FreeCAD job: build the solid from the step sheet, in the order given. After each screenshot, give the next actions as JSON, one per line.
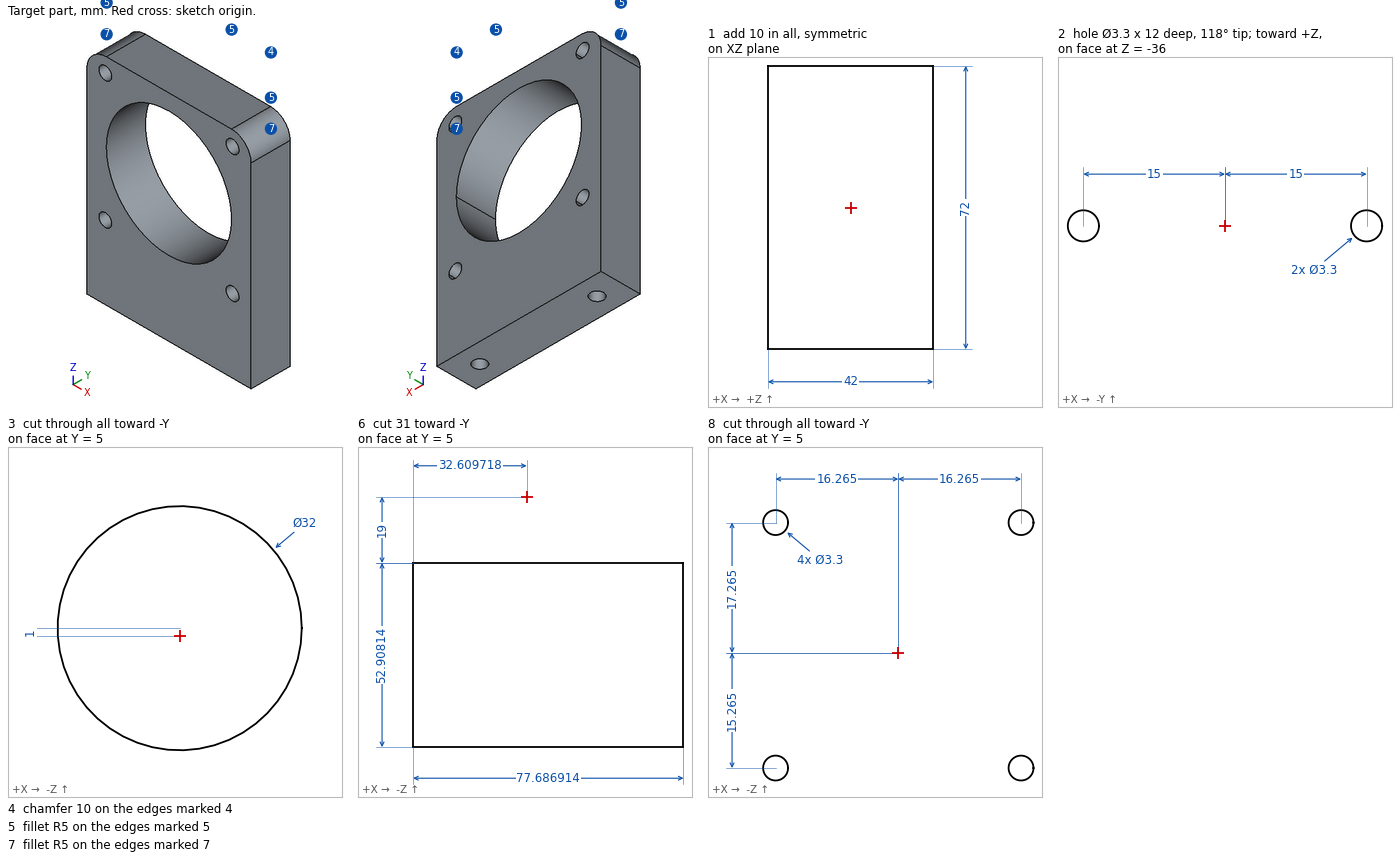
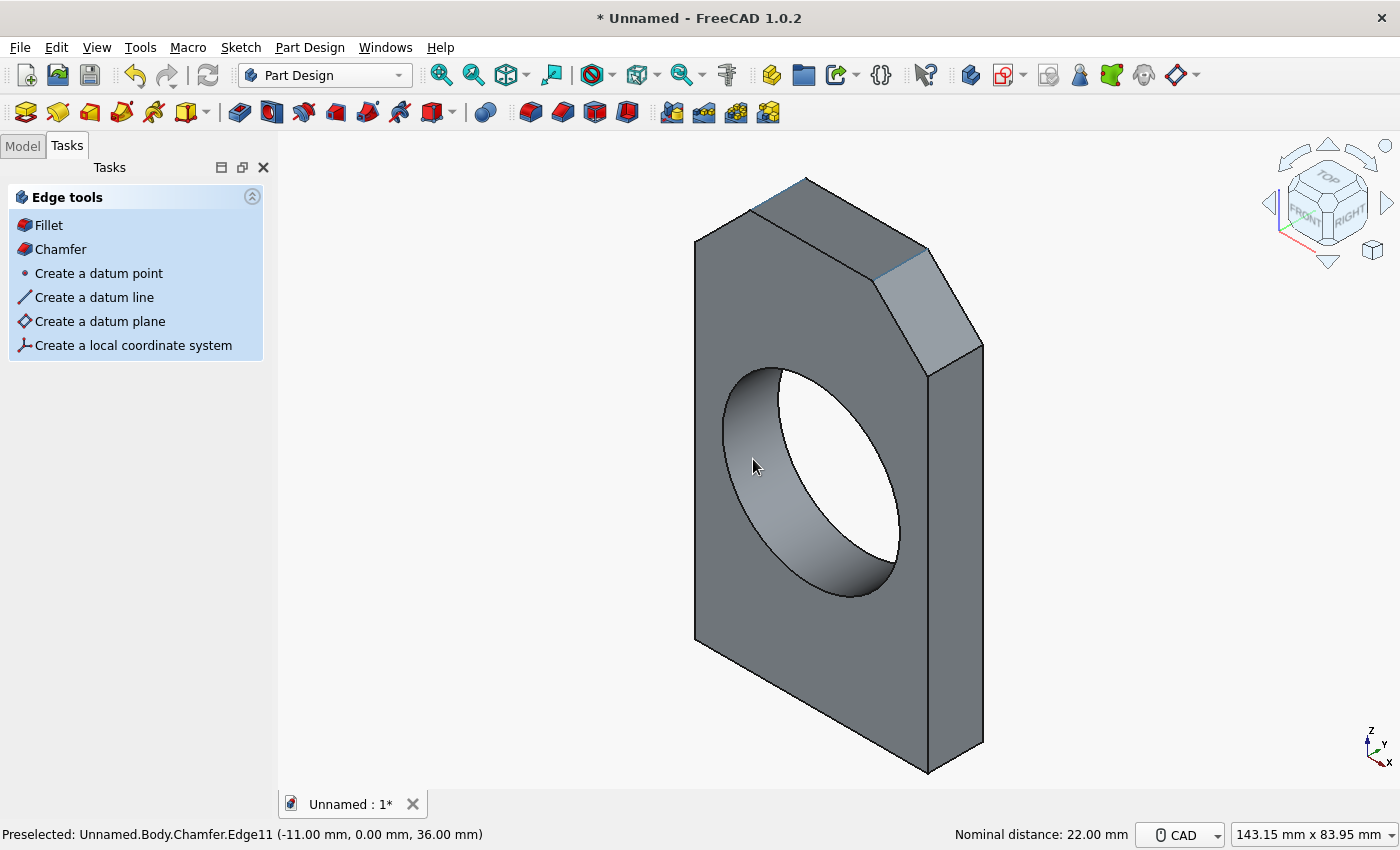
{"action": "left_click", "coordinate": [955, 360], "text": "ctrl"}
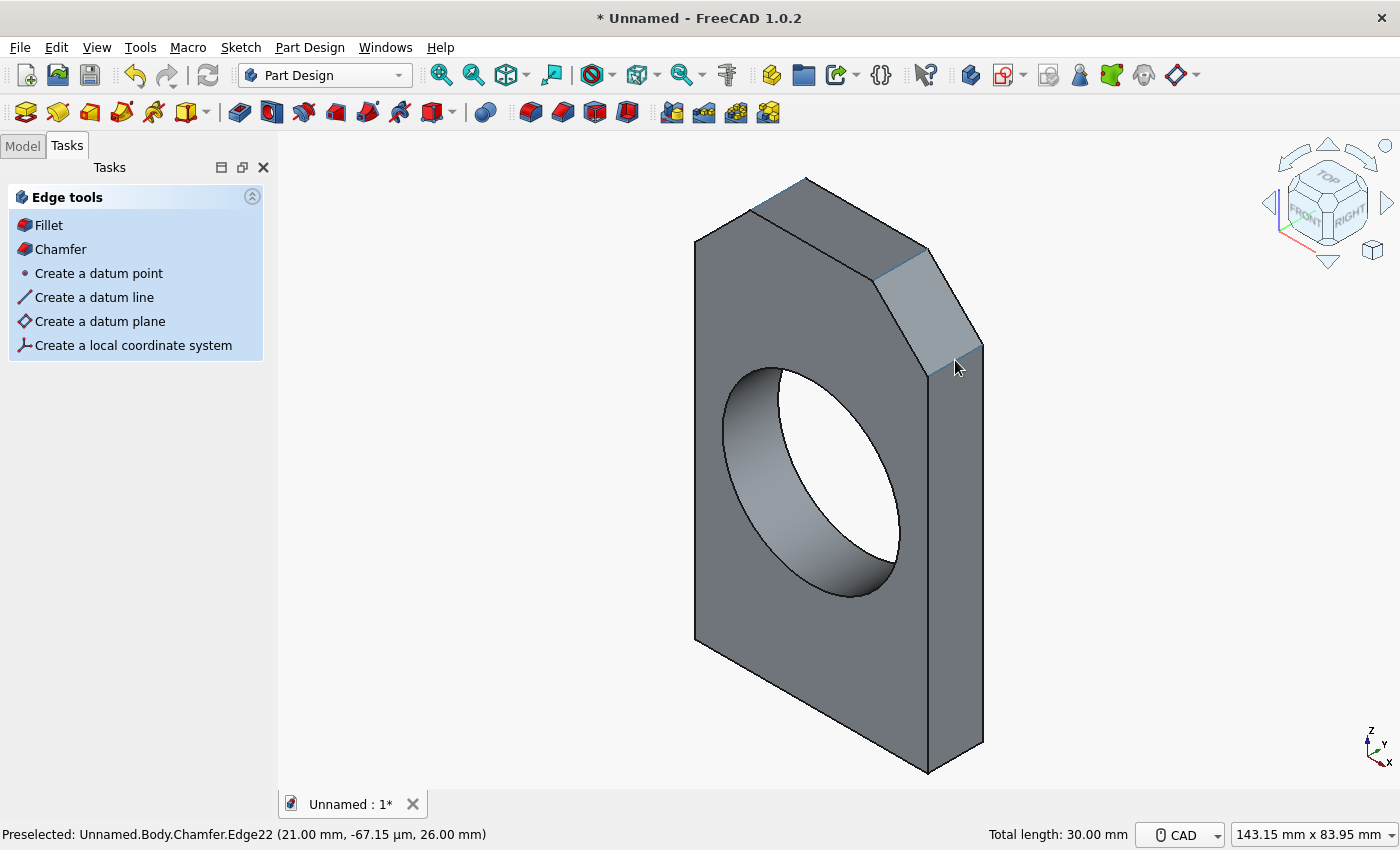
{"action": "key", "text": "2"}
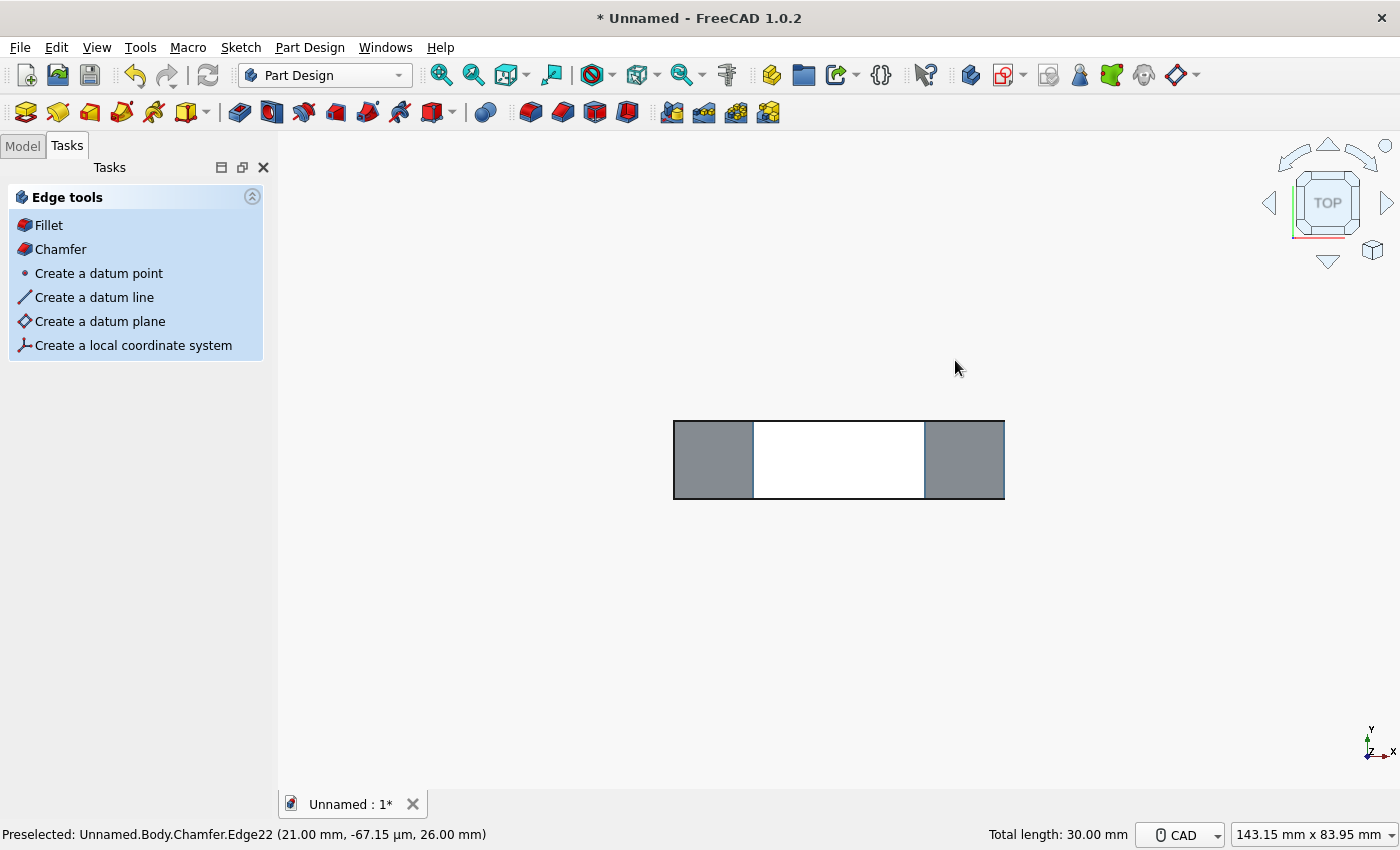
{"action": "left_click", "coordinate": [442, 76]}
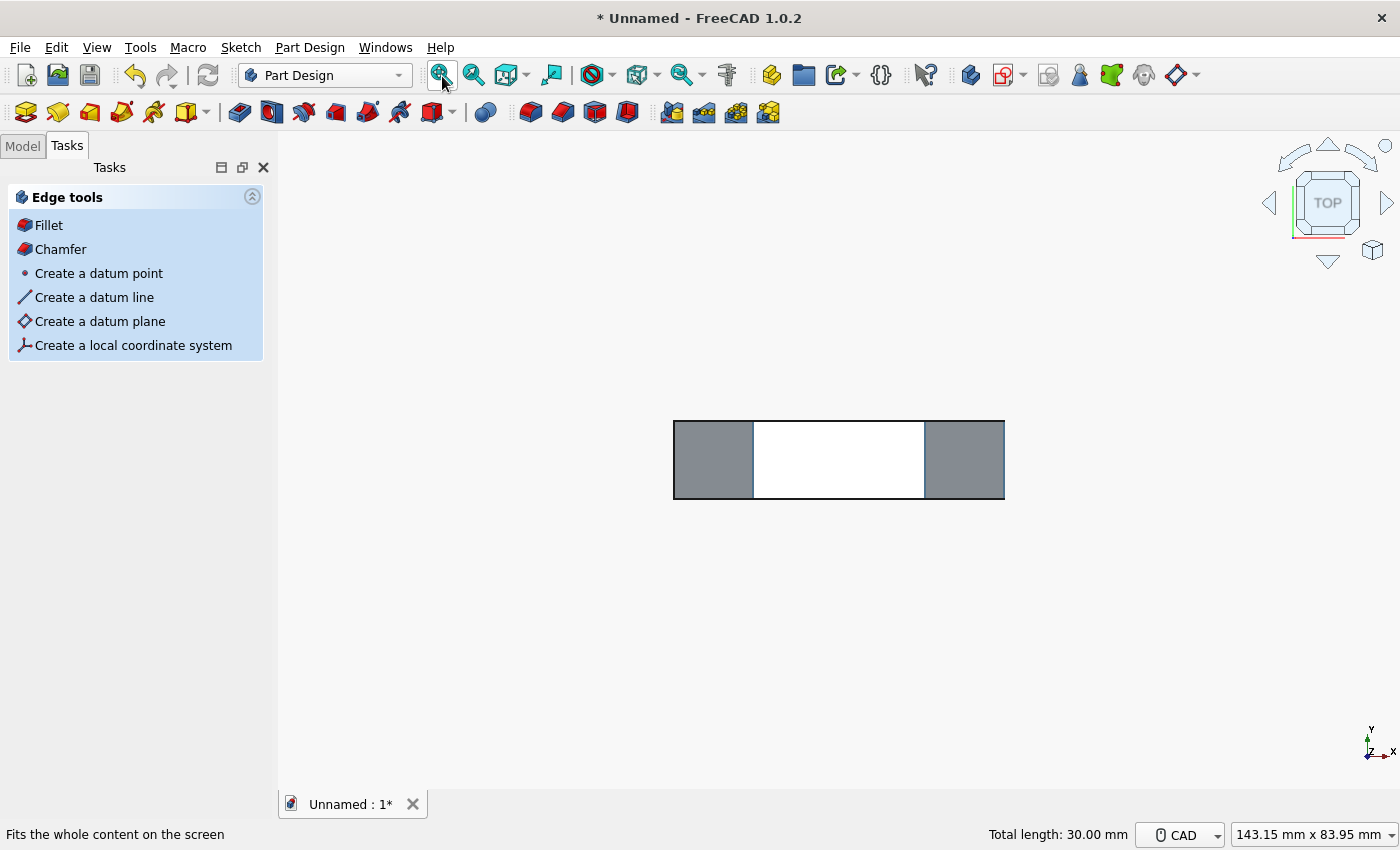
{"action": "key", "text": "1"}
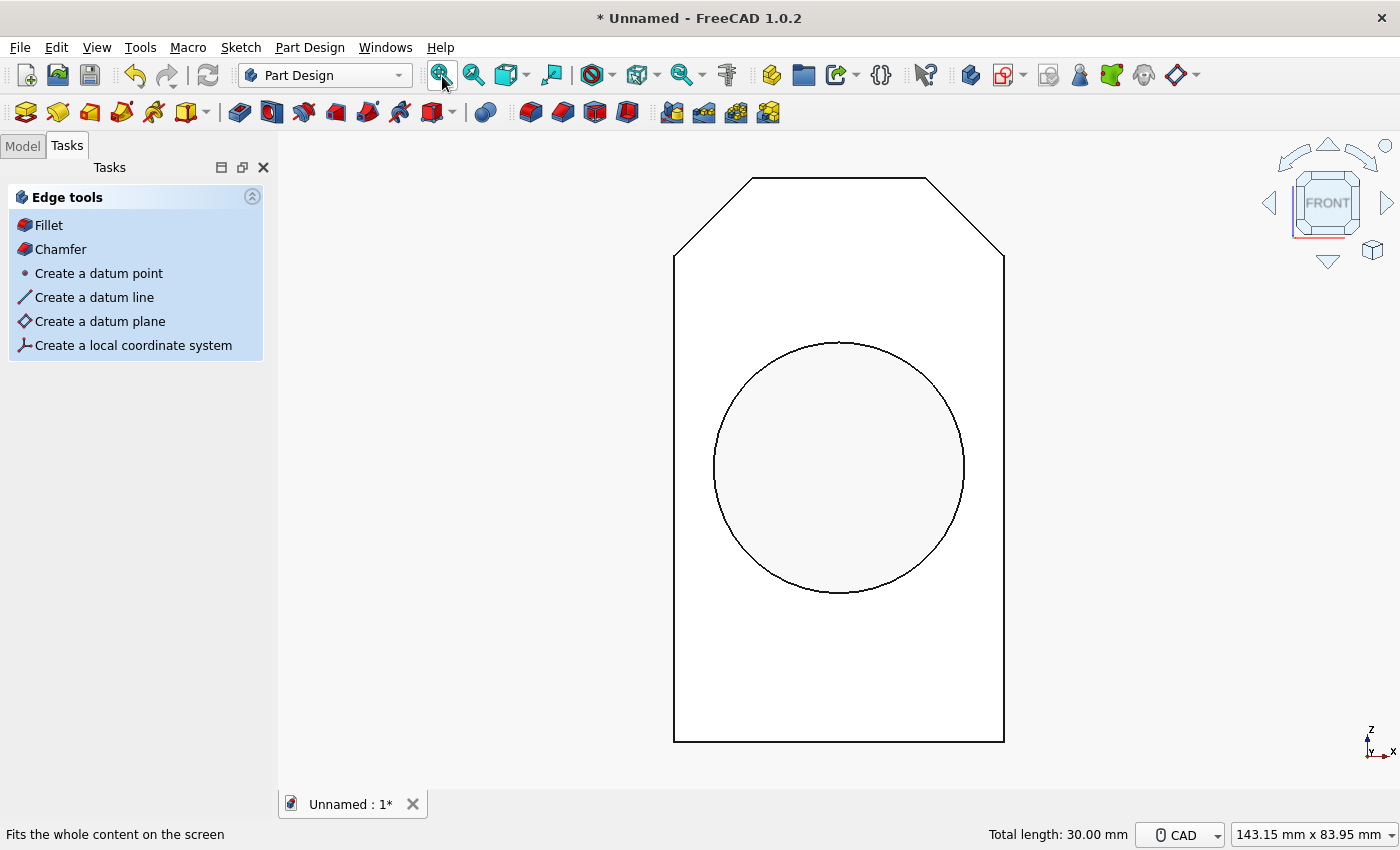
{"action": "key", "text": "3"}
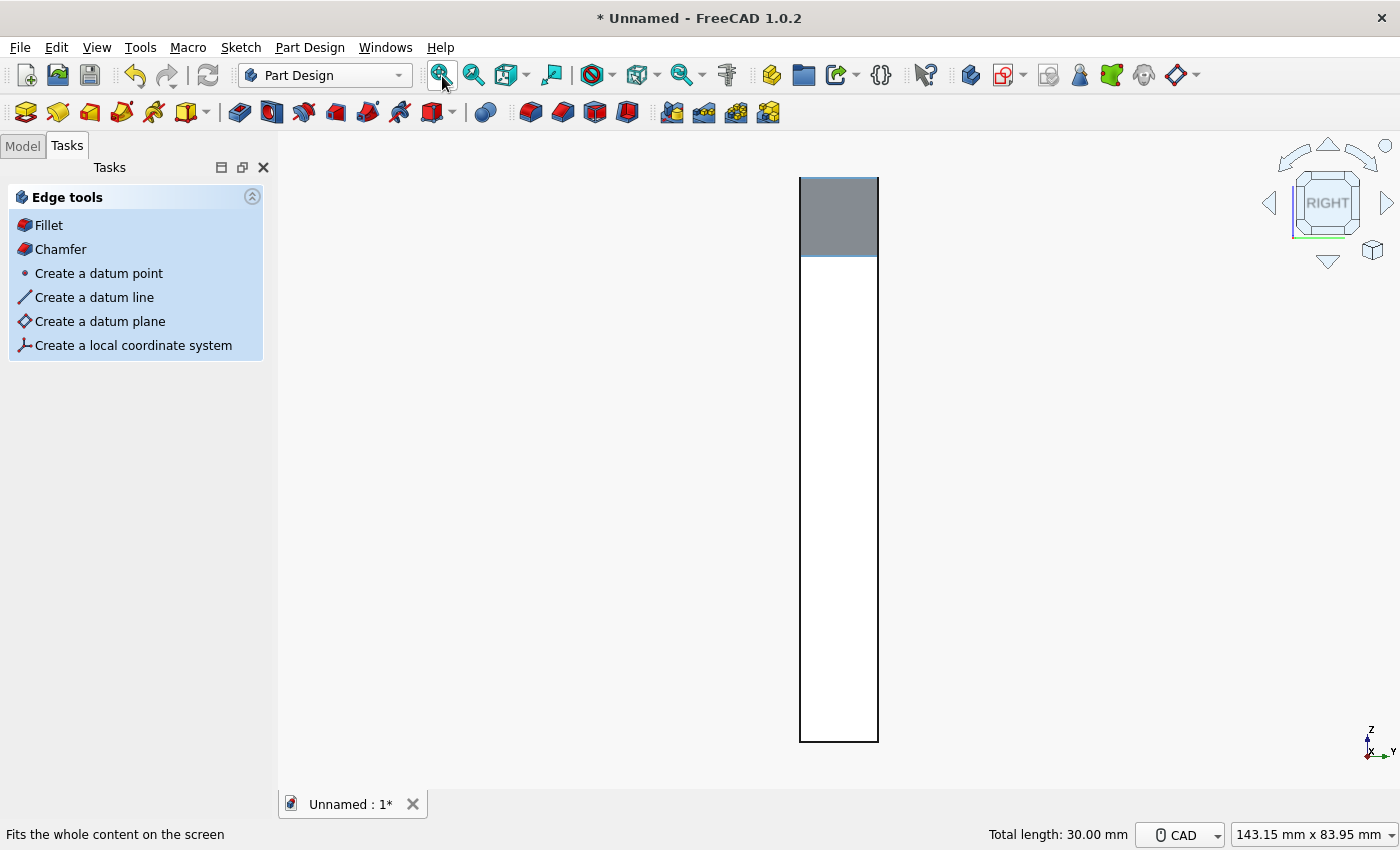
{"action": "key", "text": "5"}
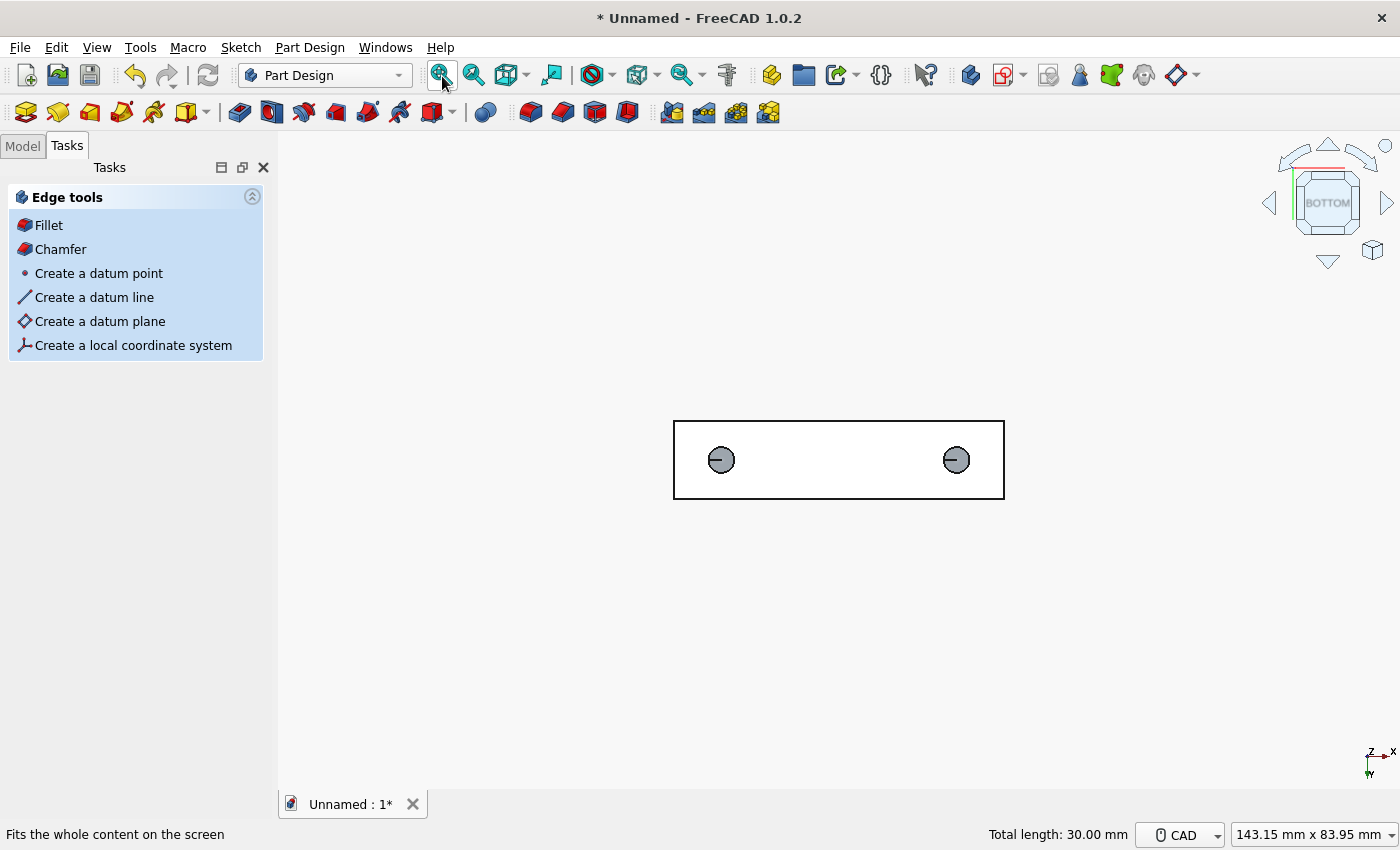
{"action": "left_click", "coordinate": [442, 76]}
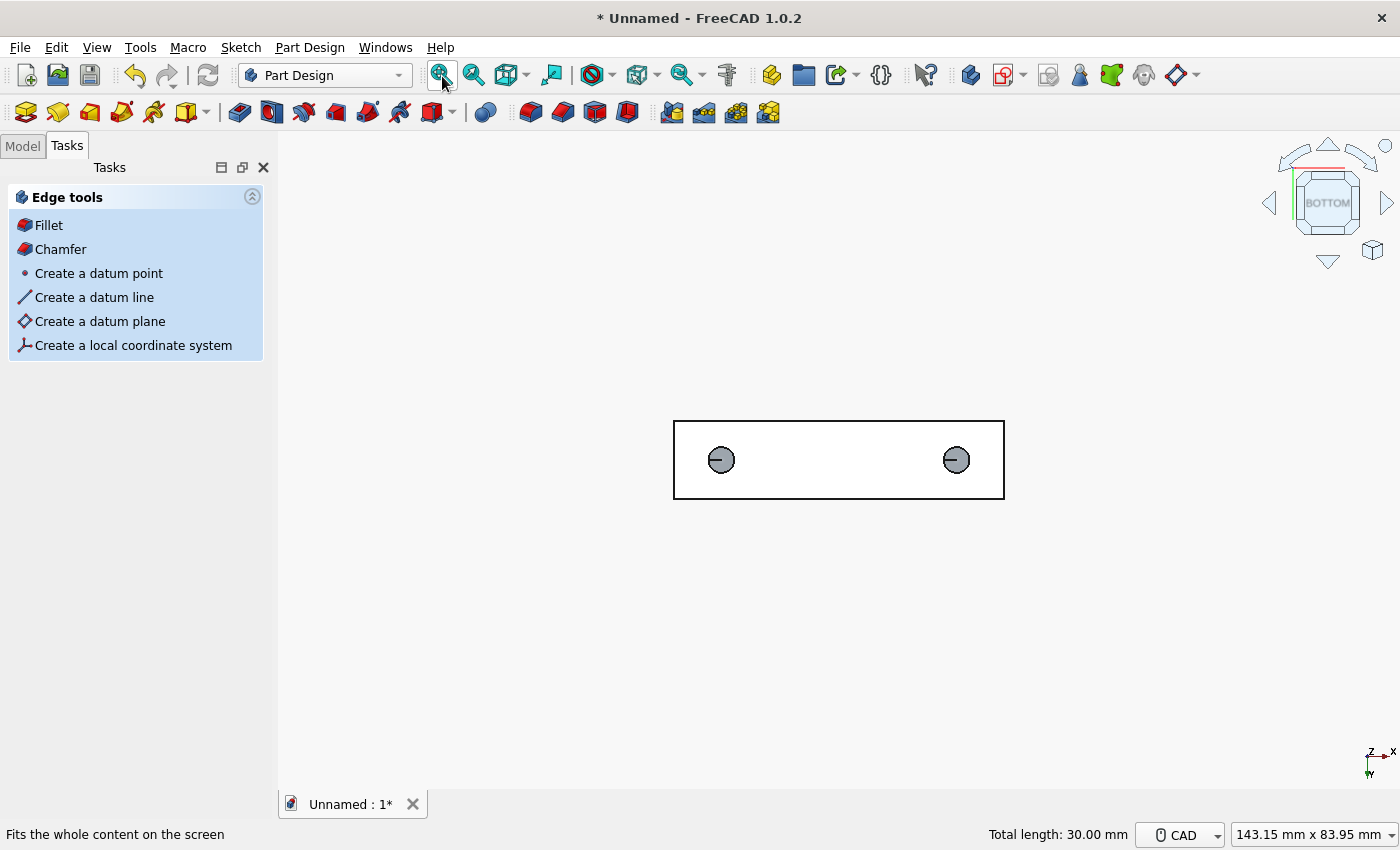
{"action": "key", "text": "4"}